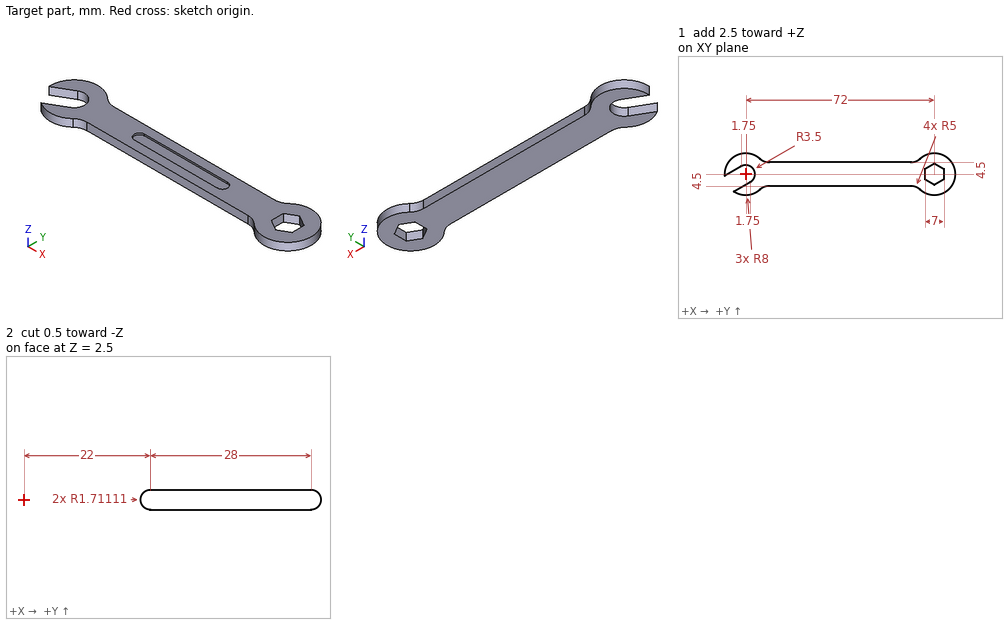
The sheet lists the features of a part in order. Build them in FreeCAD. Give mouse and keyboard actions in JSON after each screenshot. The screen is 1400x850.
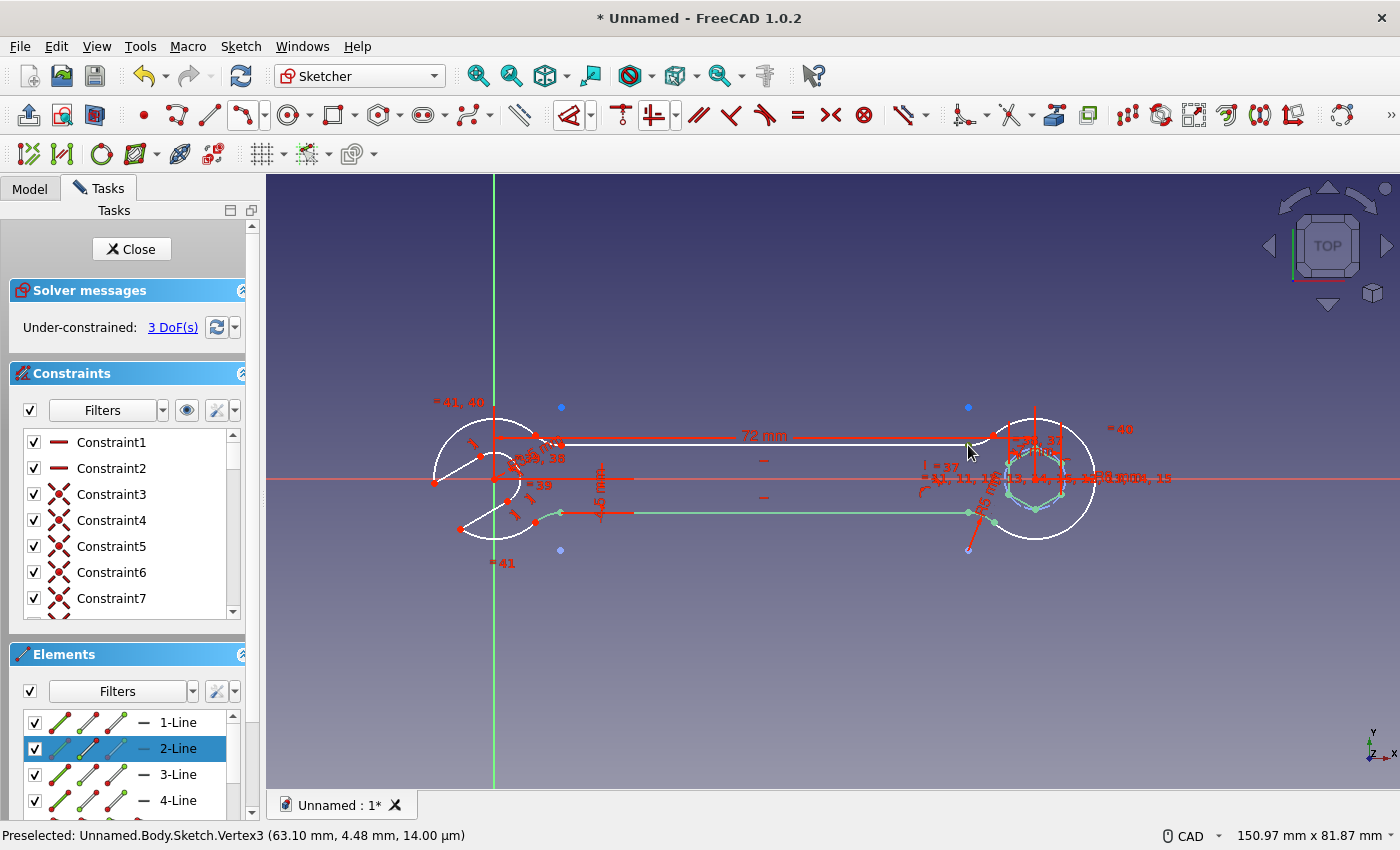
{"action": "left_click", "coordinate": [590, 116]}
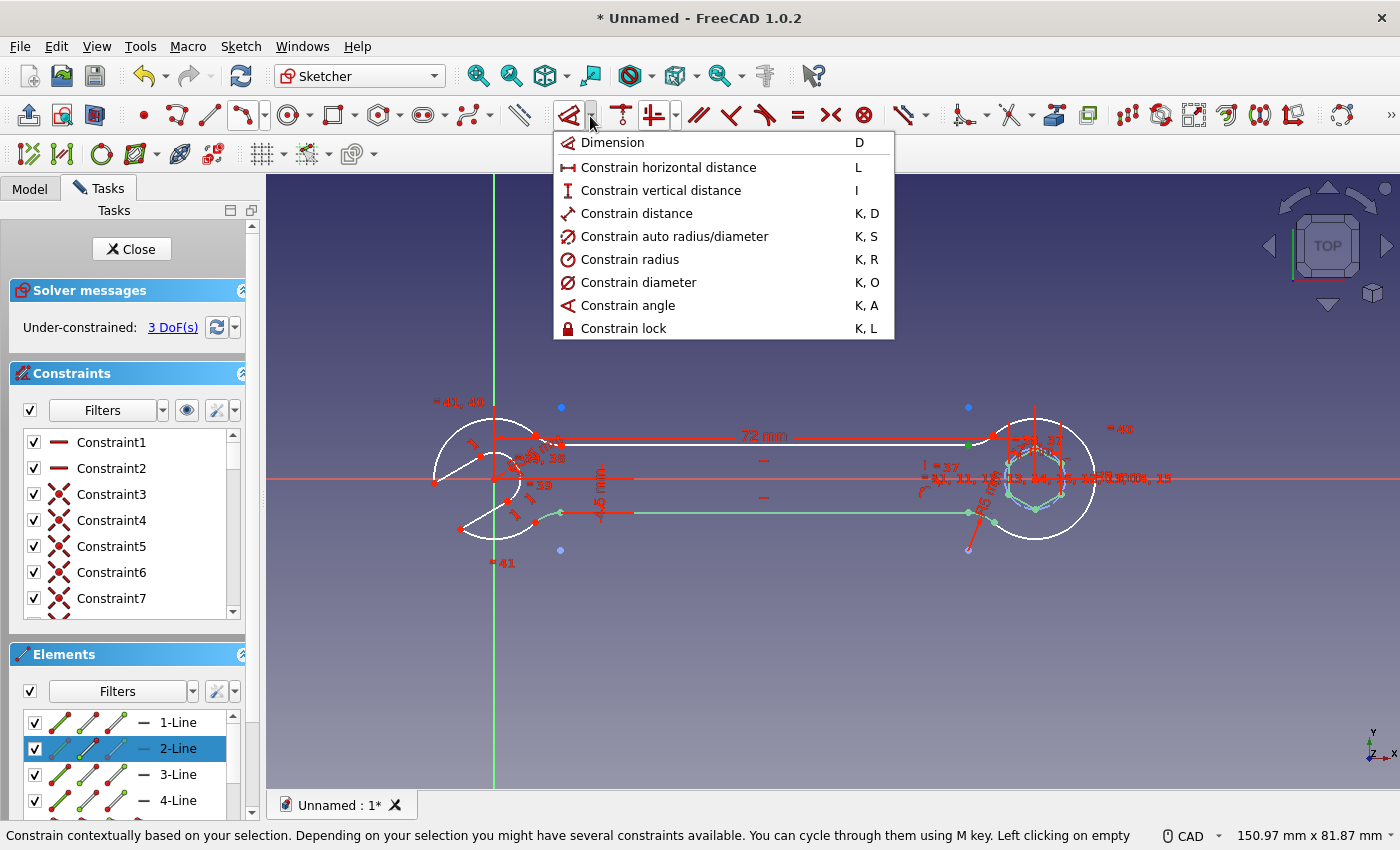
{"action": "left_click", "coordinate": [724, 190]}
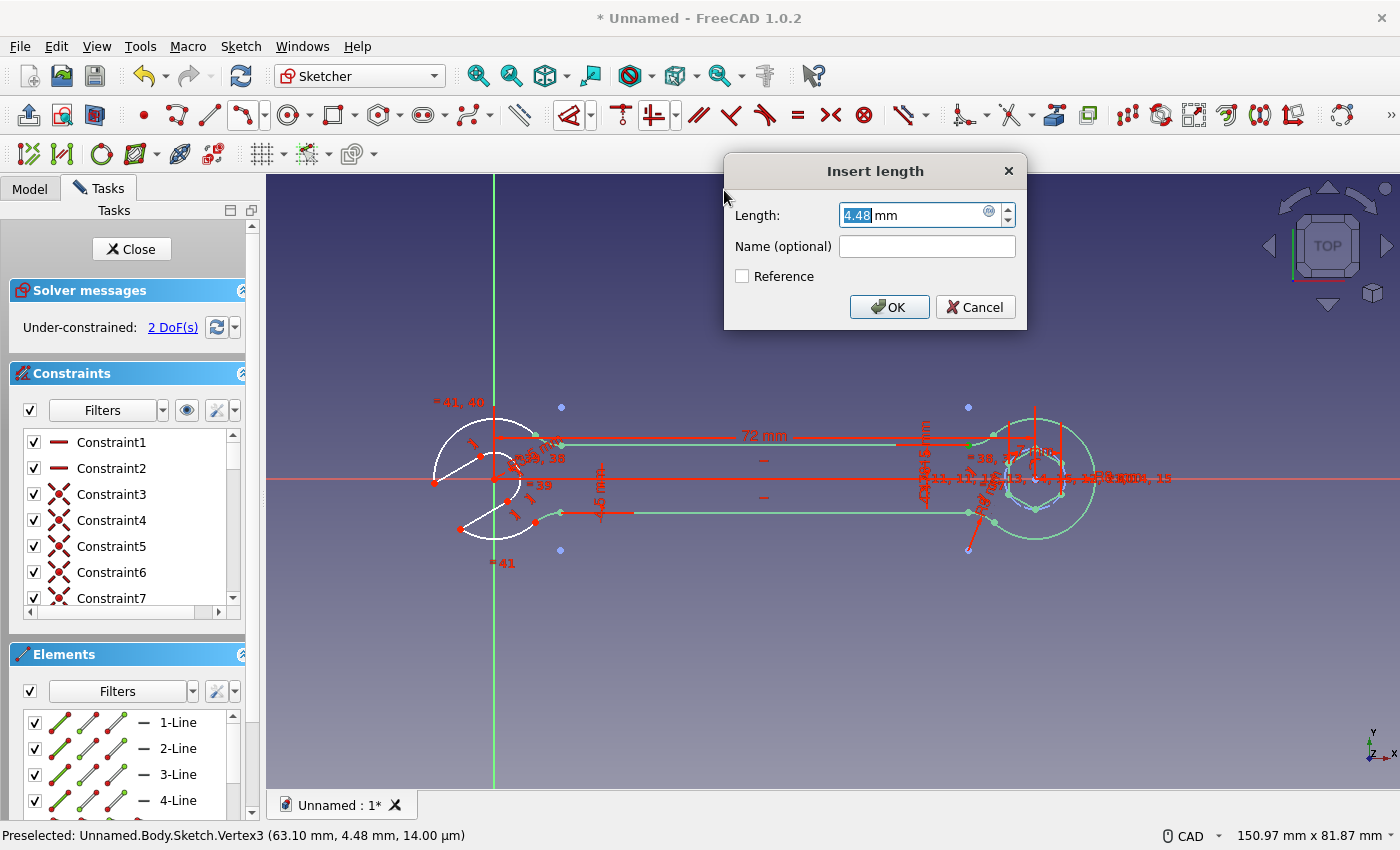
{"action": "type", "text": "4.5"}
{"action": "key", "text": "Return"}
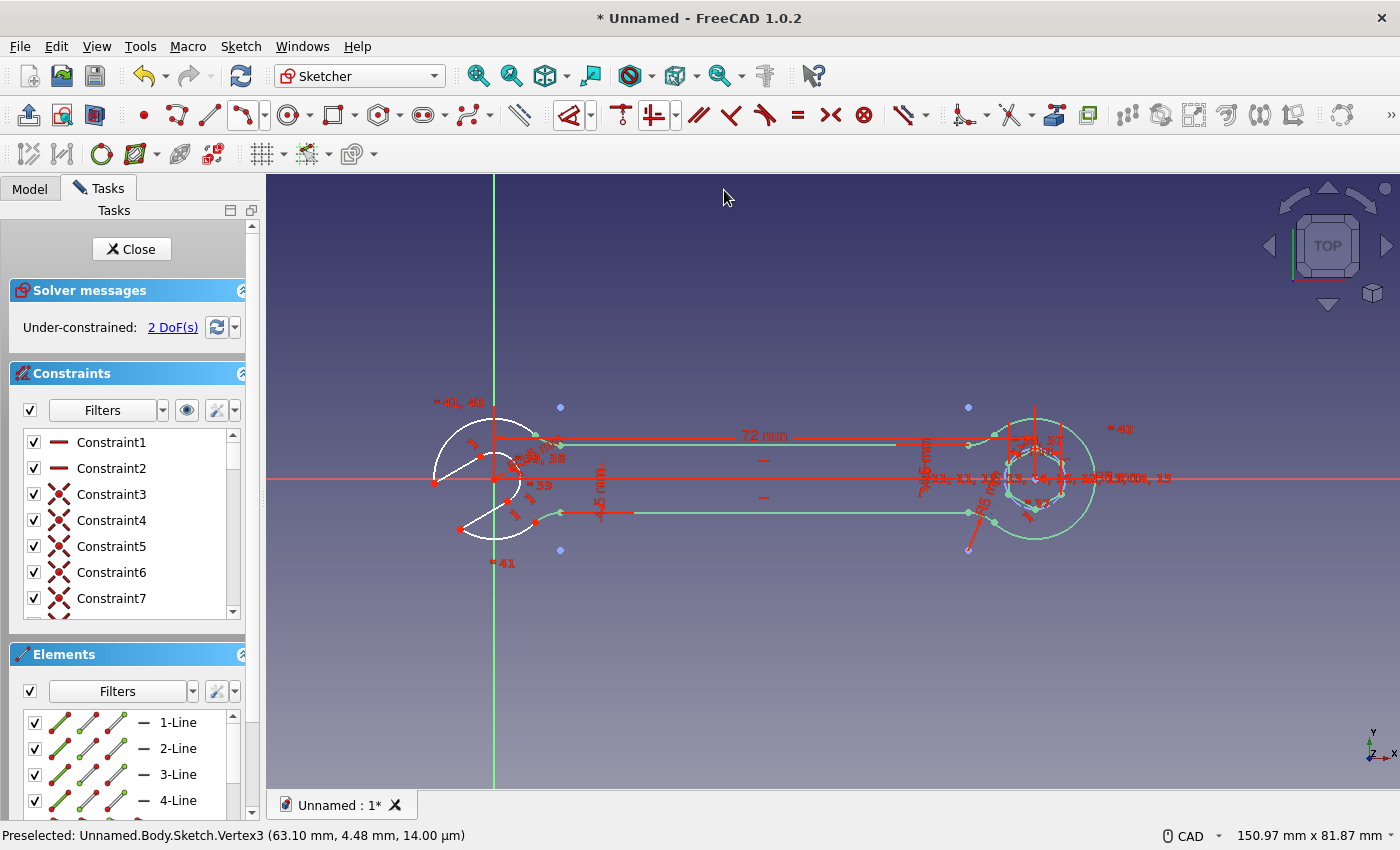
{"action": "scroll", "coordinate": [481, 456], "scroll_direction": "up", "scroll_amount": 6}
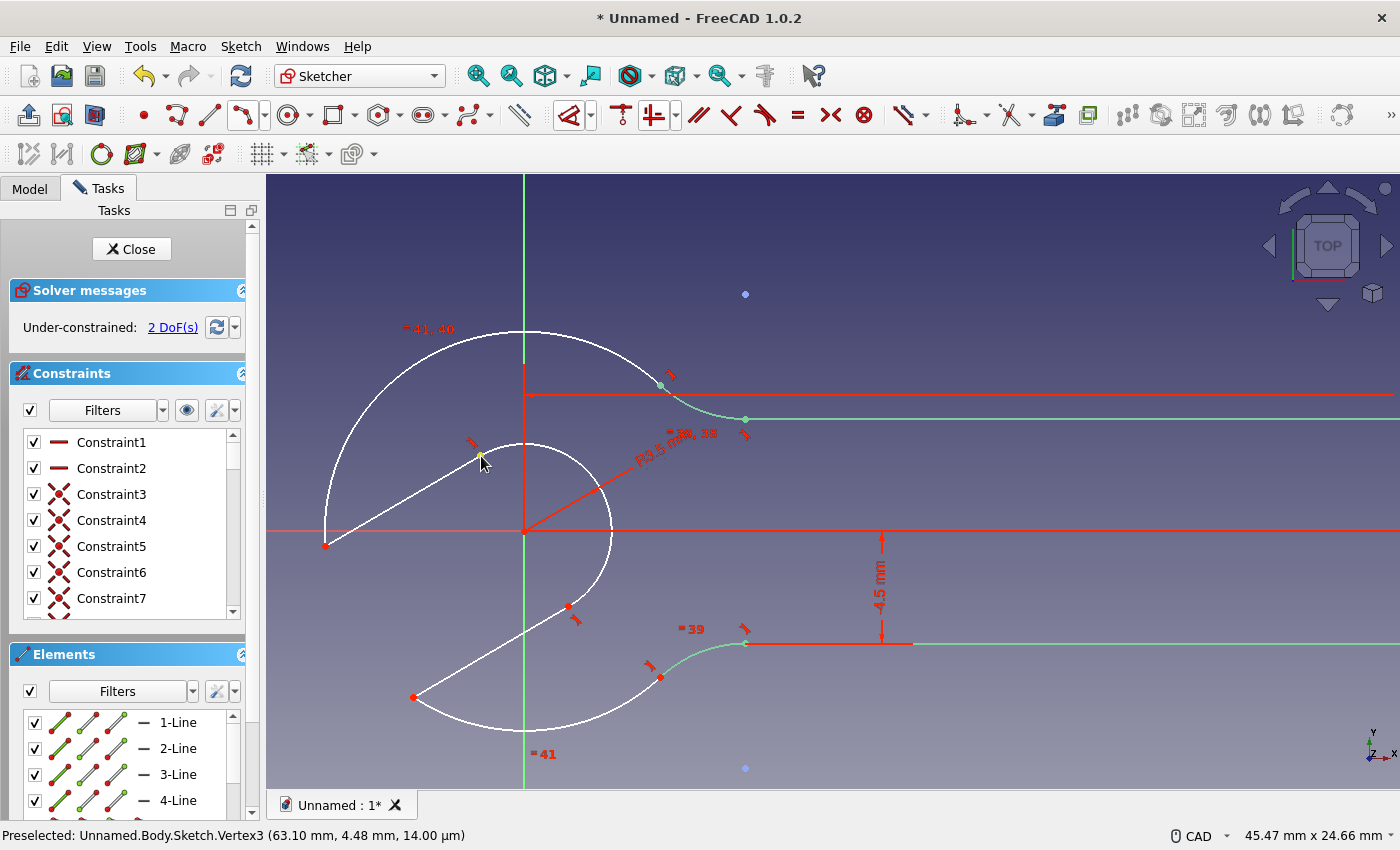
{"action": "left_click", "coordinate": [480, 456]}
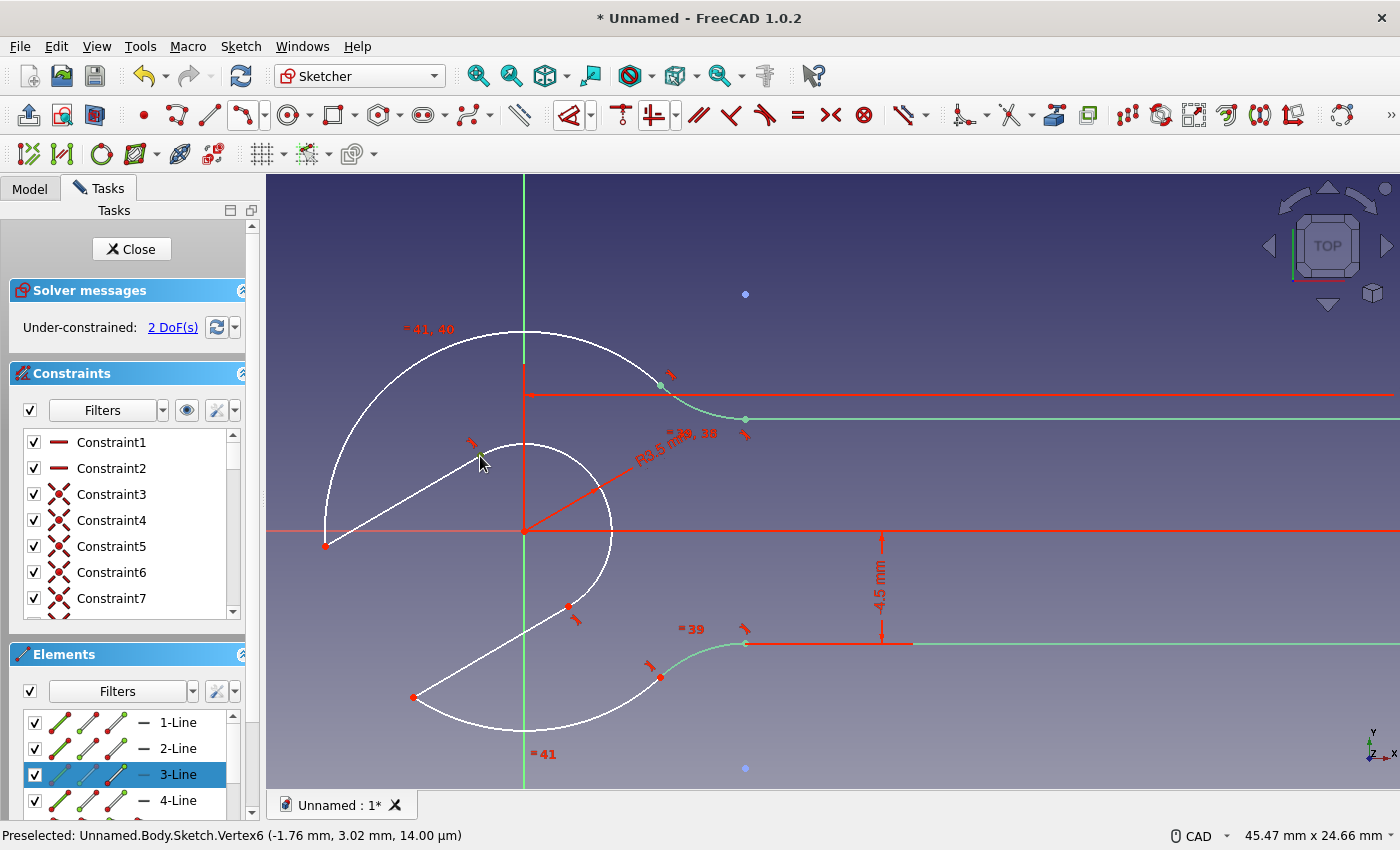
{"action": "left_click", "coordinate": [590, 116]}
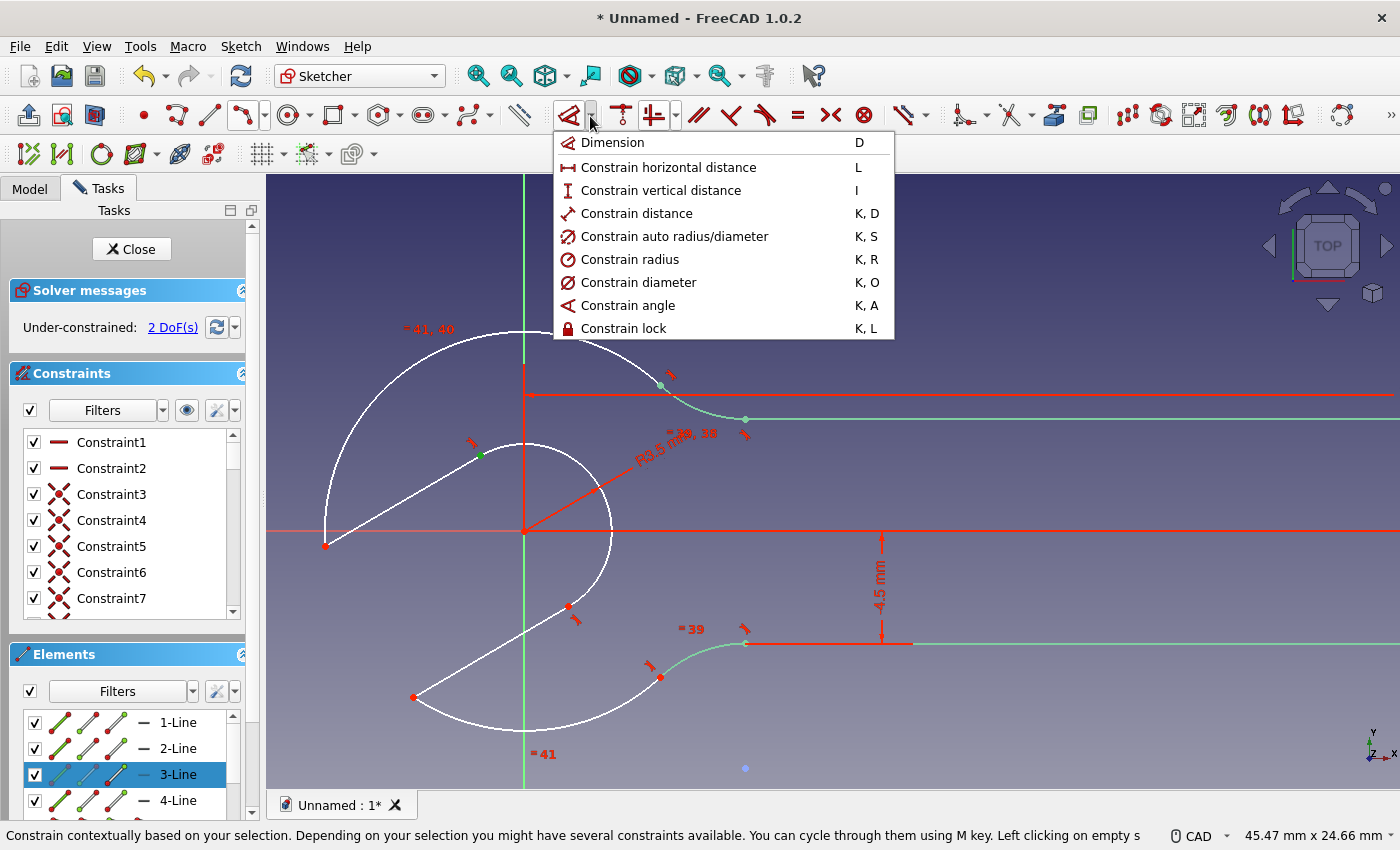
{"action": "left_click", "coordinate": [724, 168]}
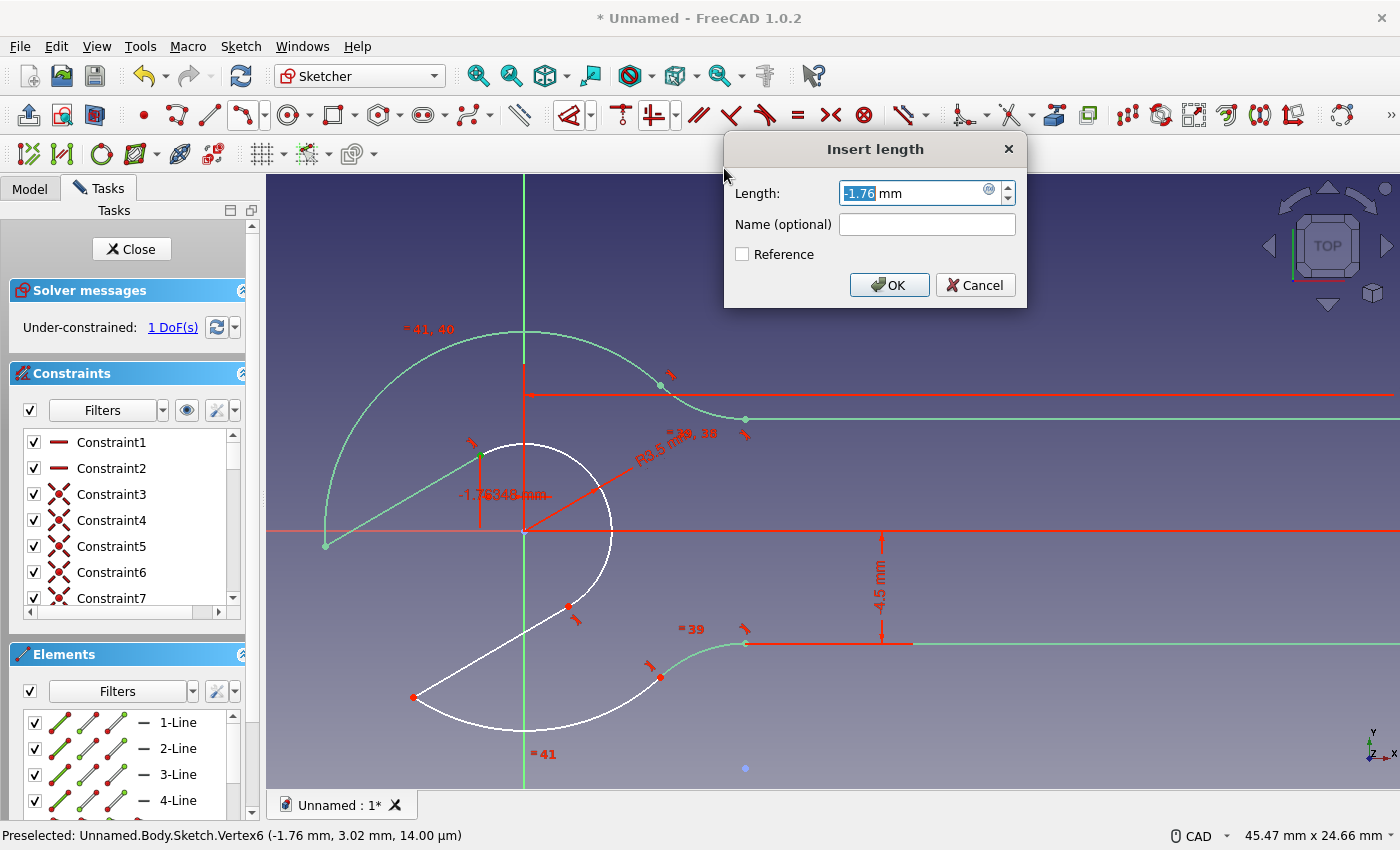
{"action": "type", "text": "-1.75"}
{"action": "key", "text": "Return"}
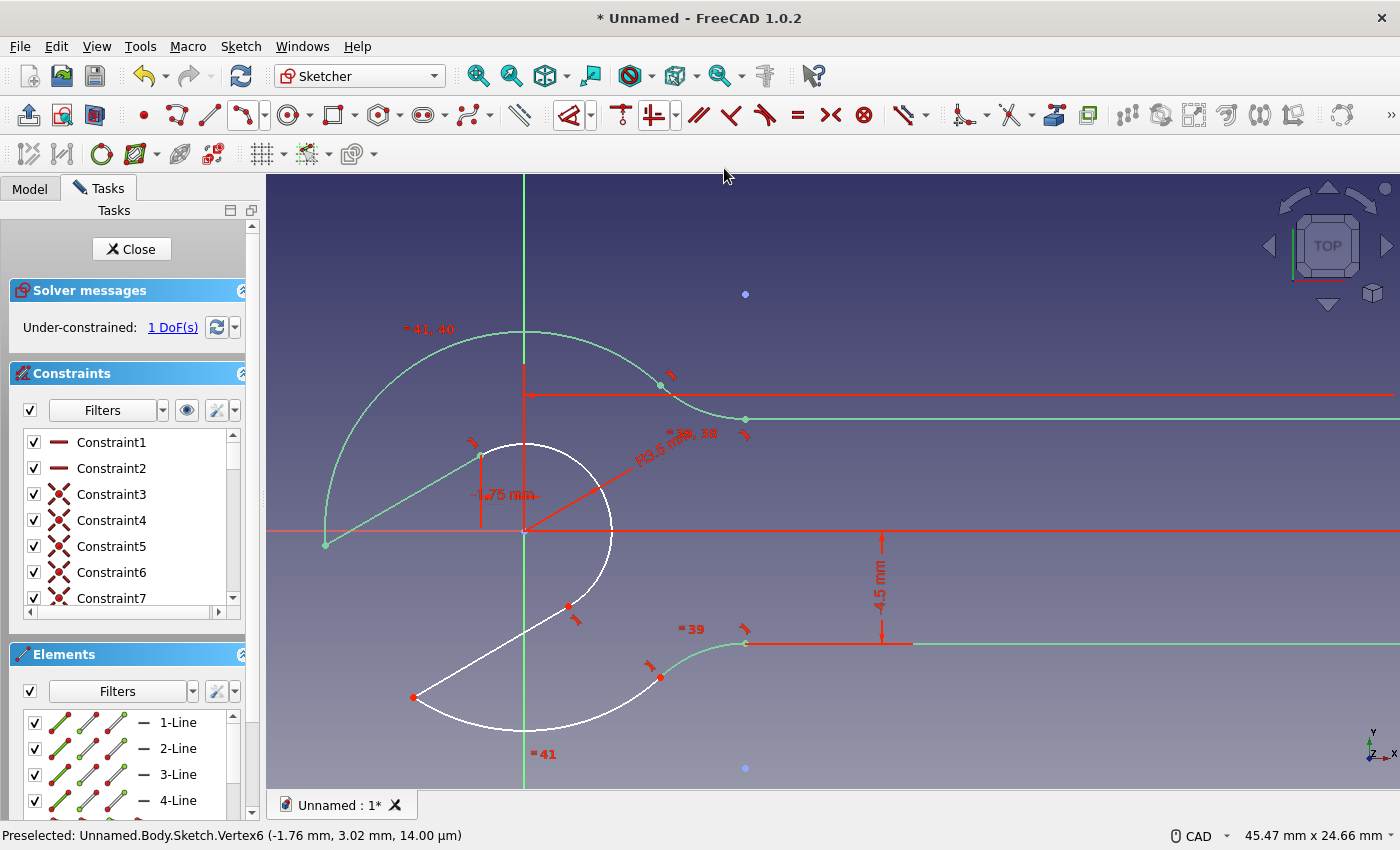
{"action": "left_click", "coordinate": [569, 607]}